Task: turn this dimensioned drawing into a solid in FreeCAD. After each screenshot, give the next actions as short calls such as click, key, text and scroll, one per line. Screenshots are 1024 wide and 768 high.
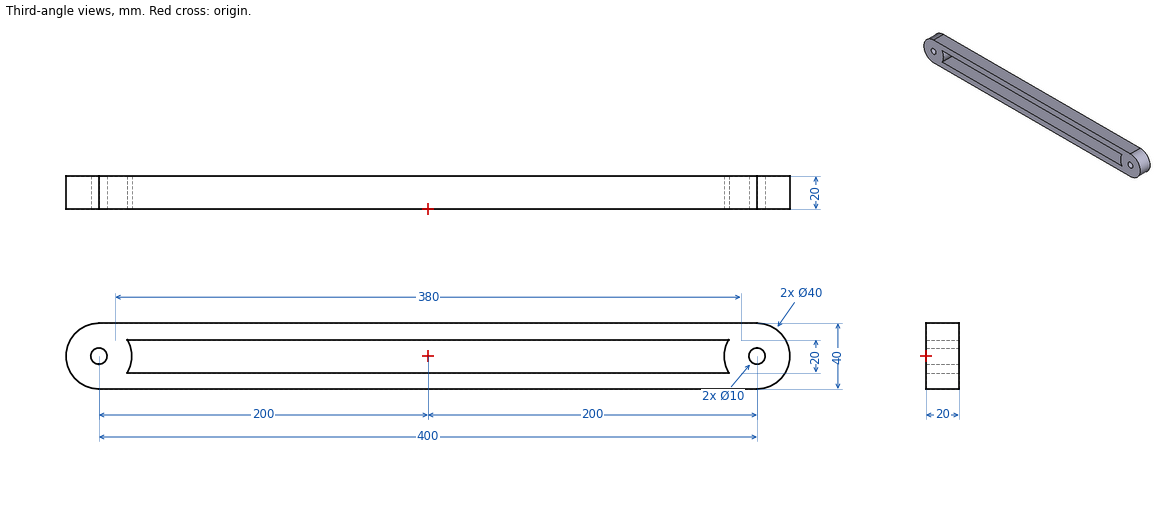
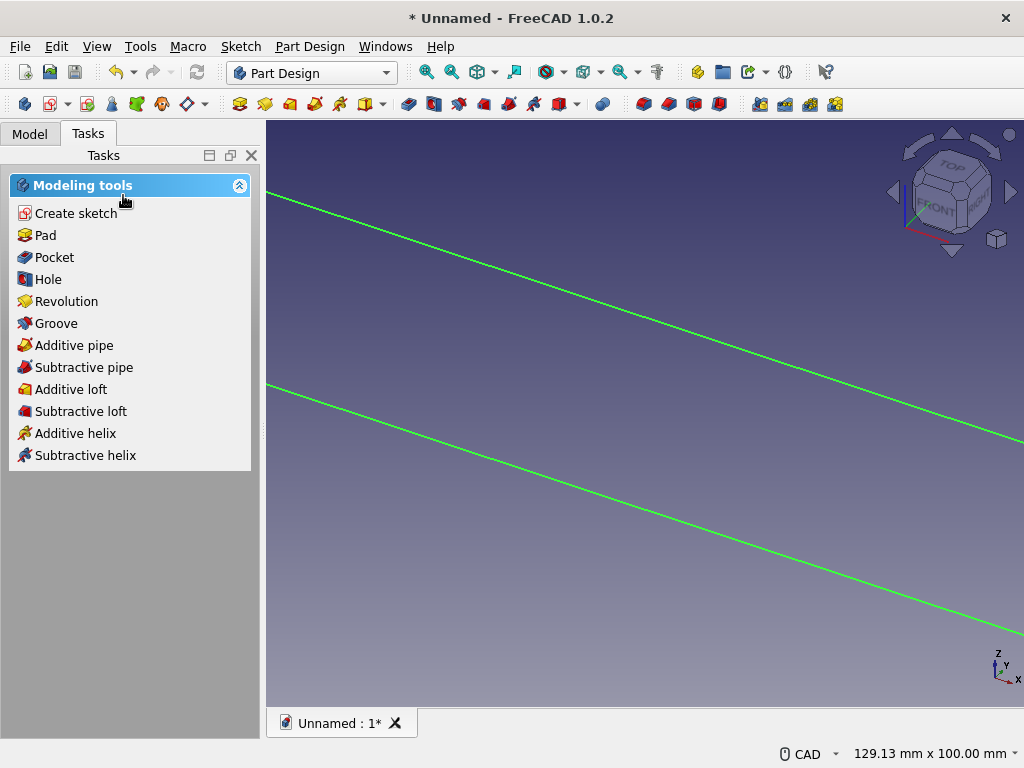
click(240, 104)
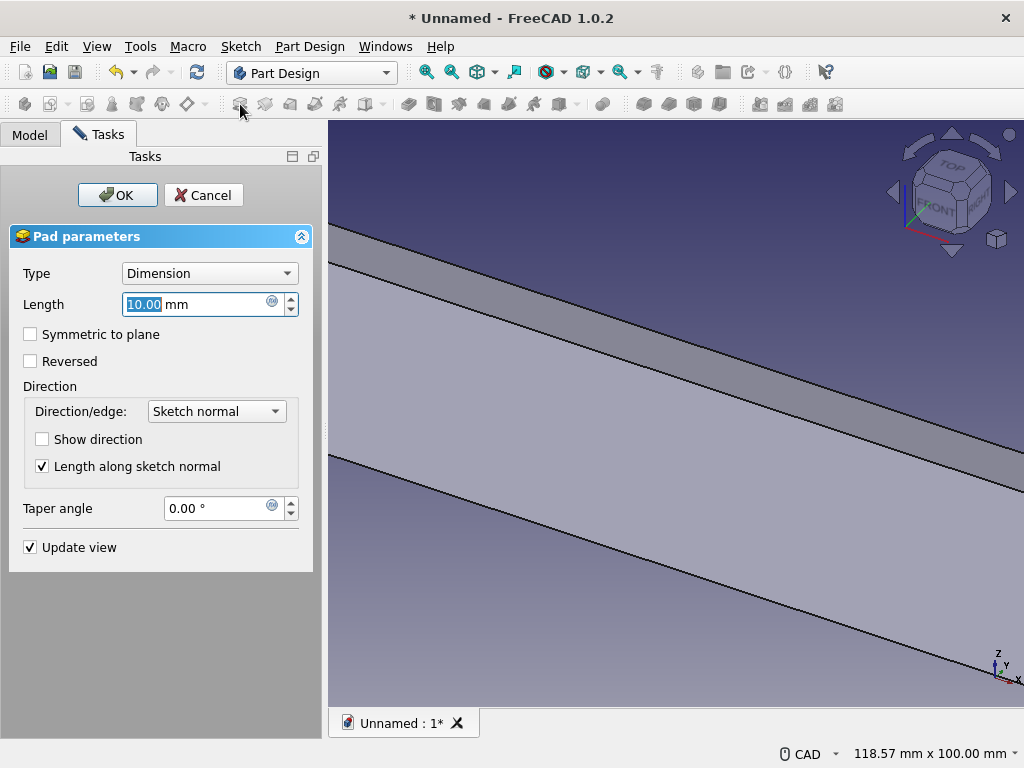
text(20)
key(Tab)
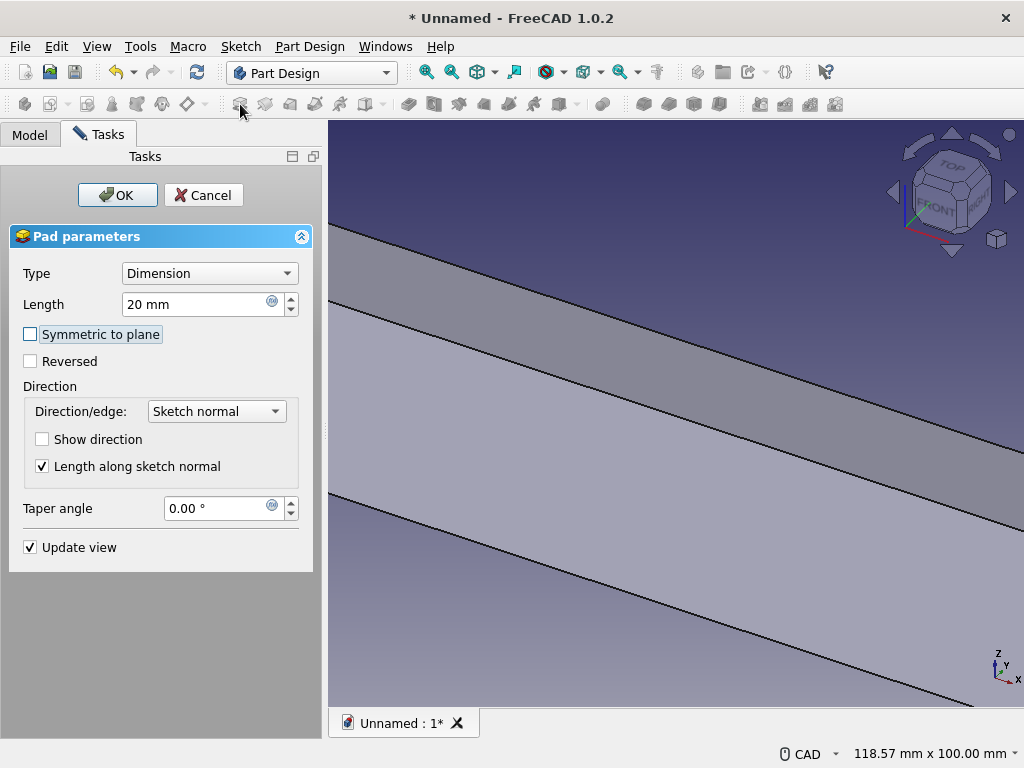
click(31, 361)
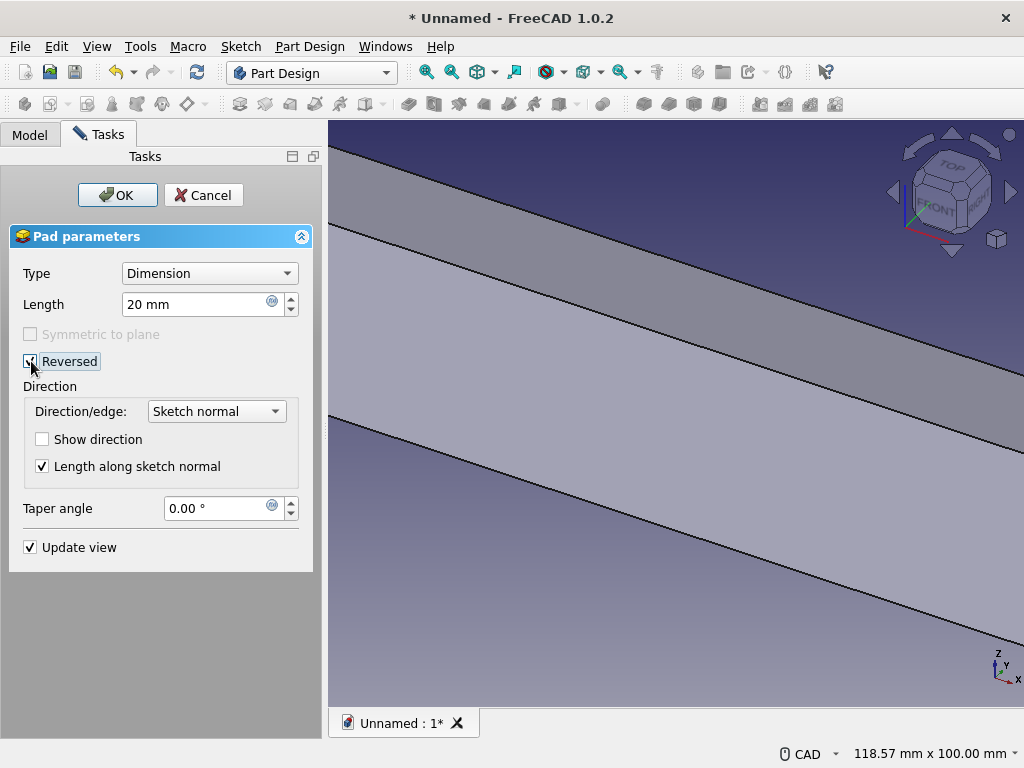
click(118, 195)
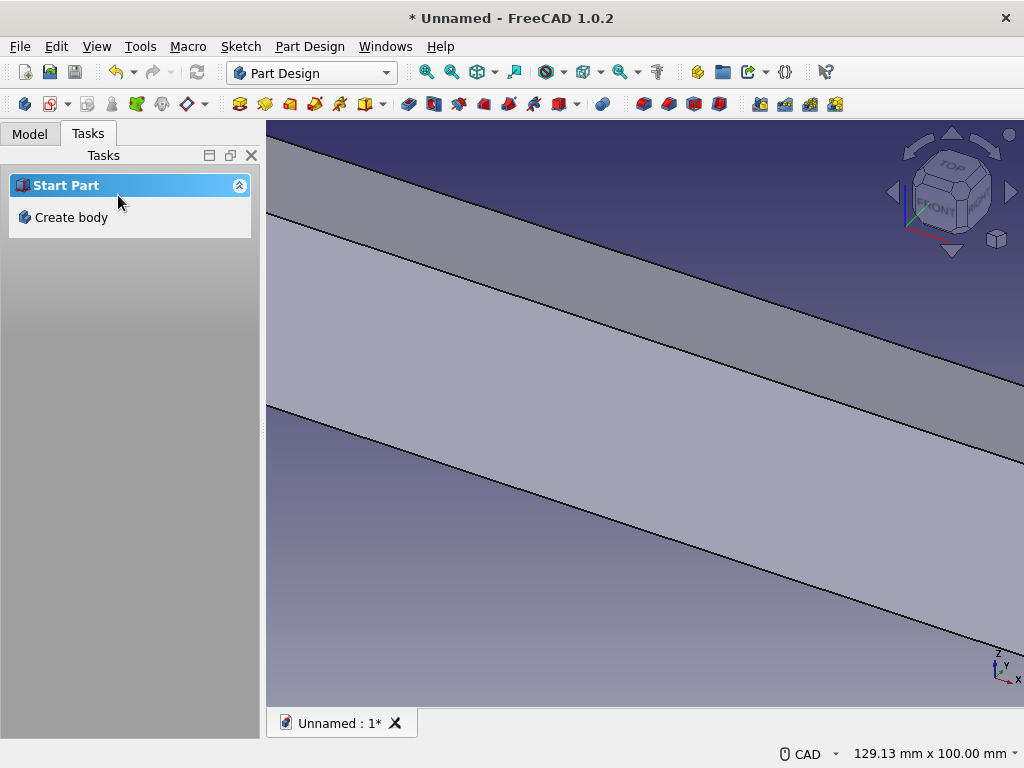
click(427, 72)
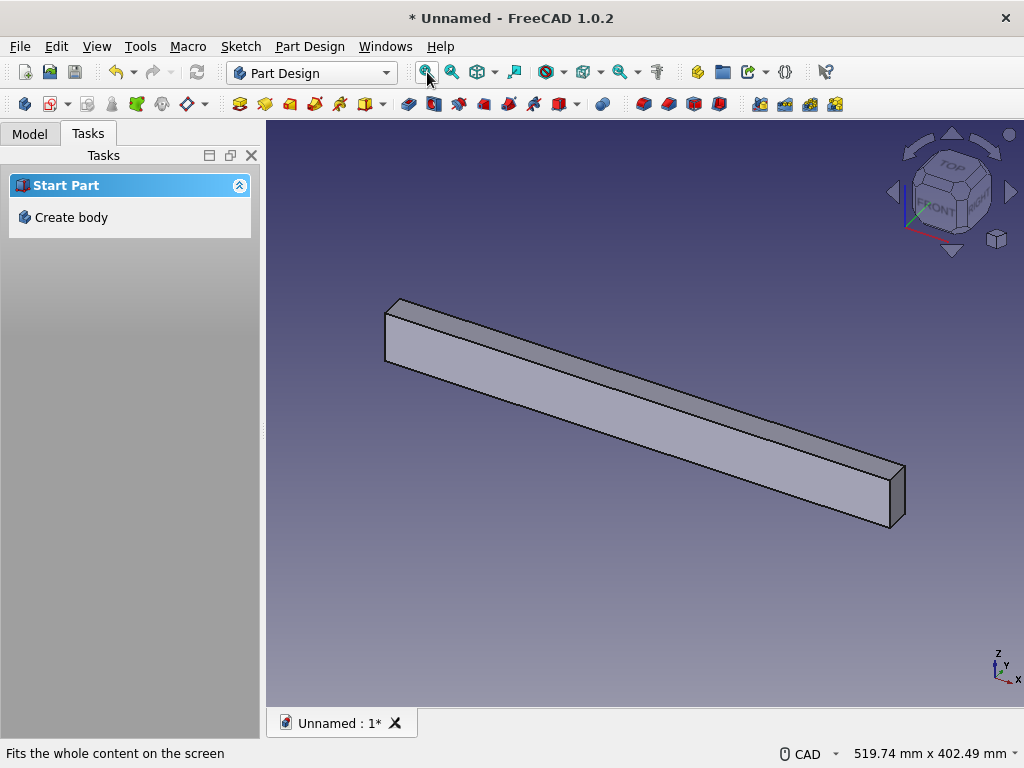
key(4)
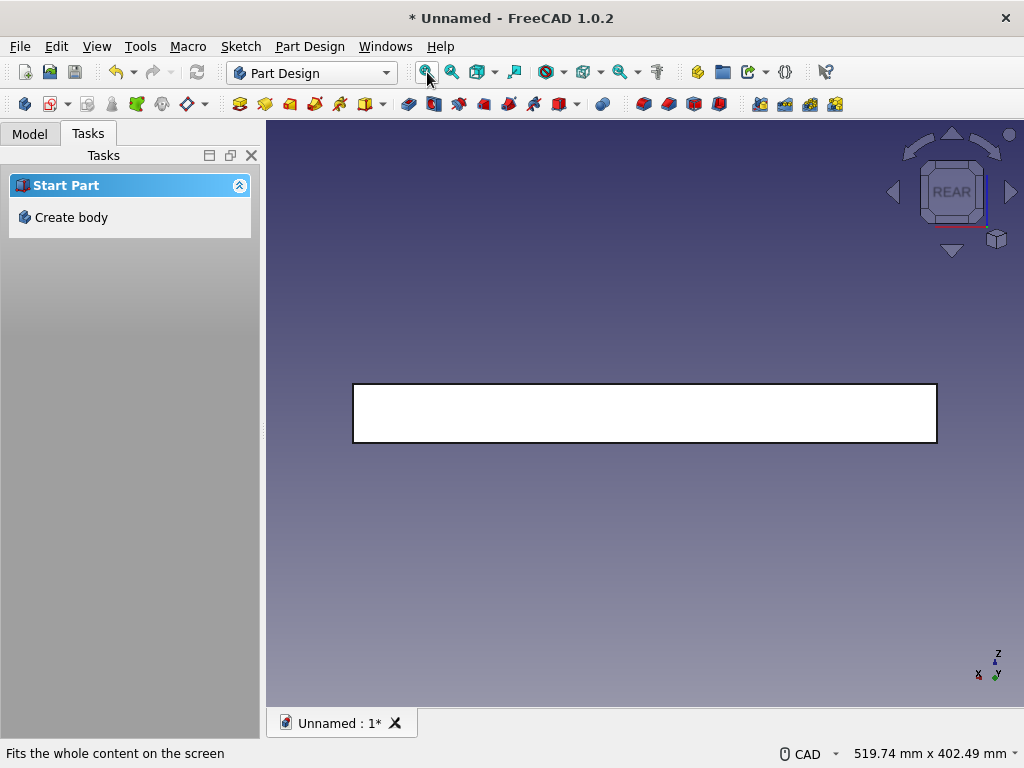
click(395, 413)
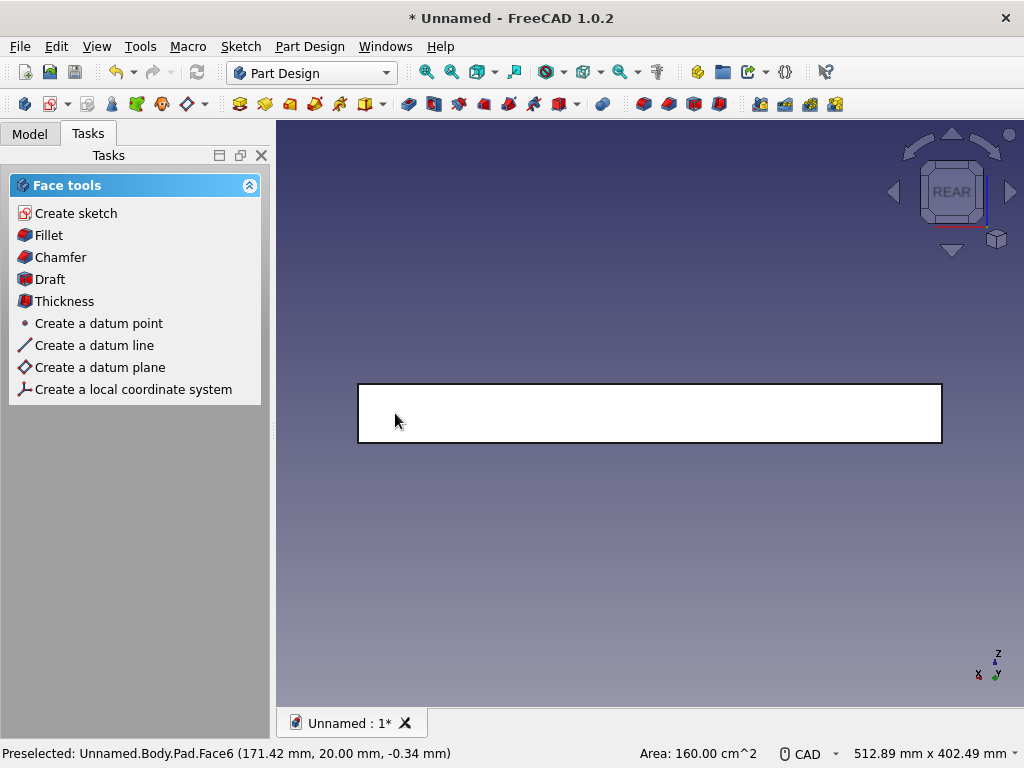
click(50, 104)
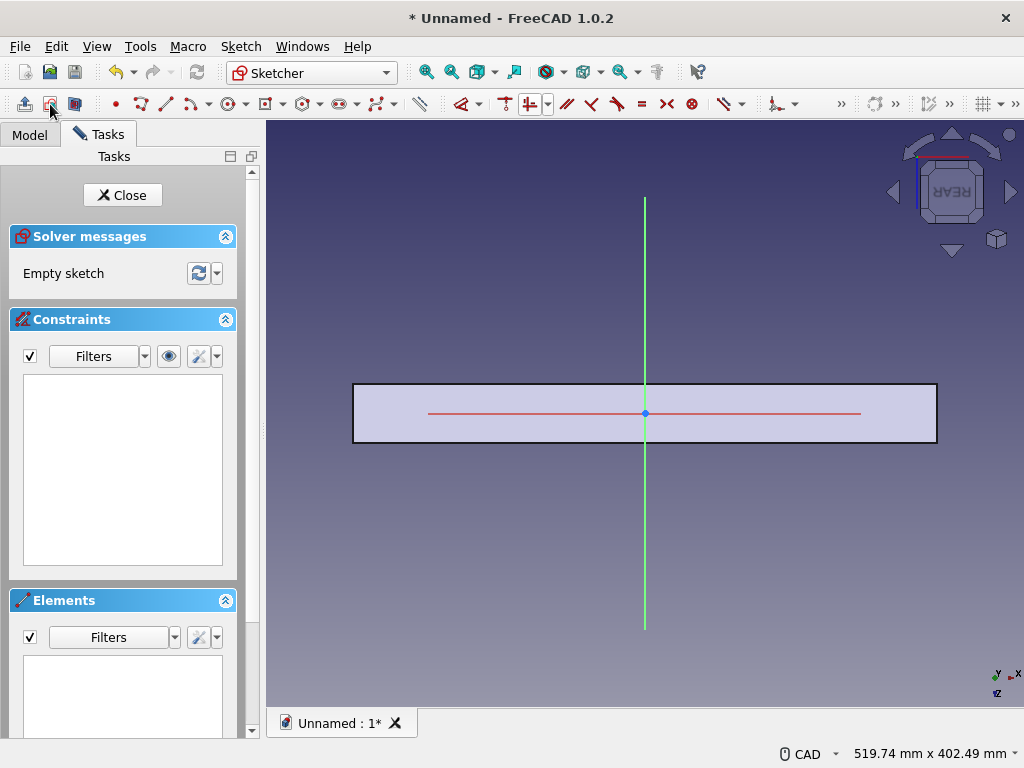
scroll(437, 414, down, 2)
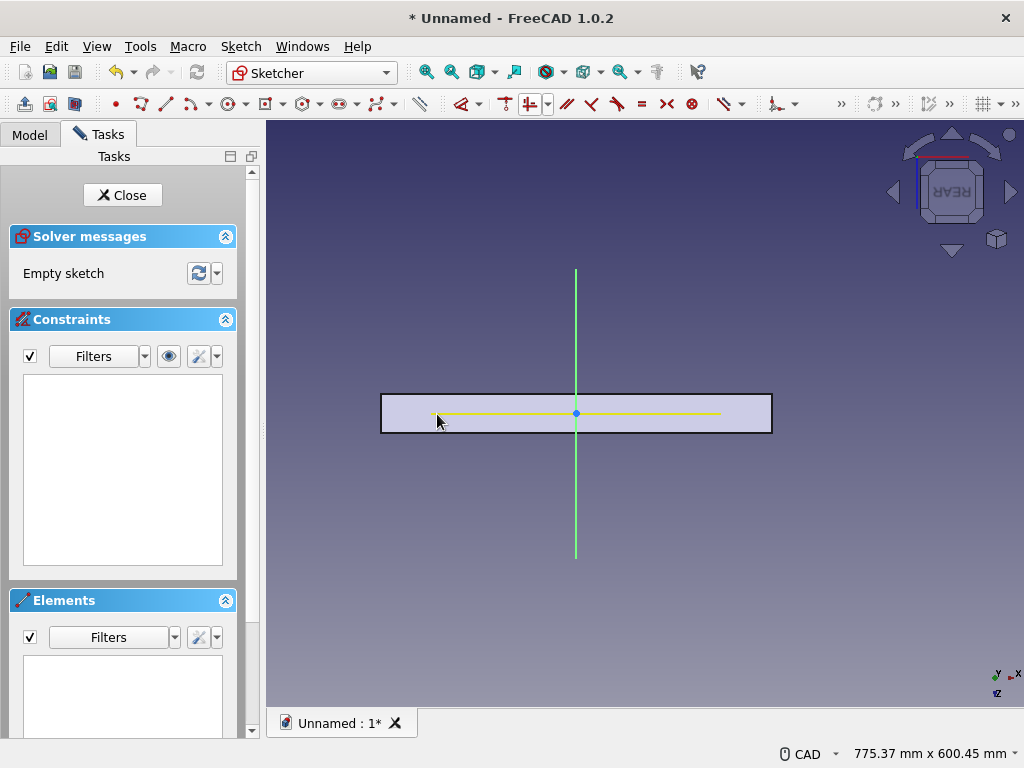
click(264, 104)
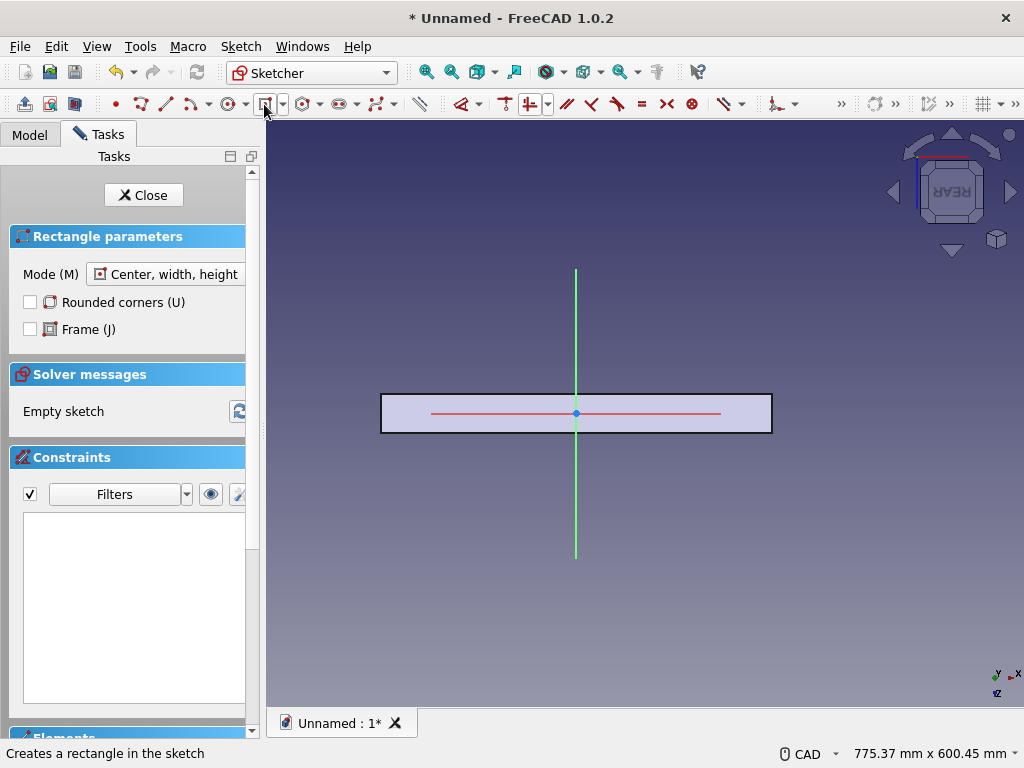
scroll(577, 414, up, 3)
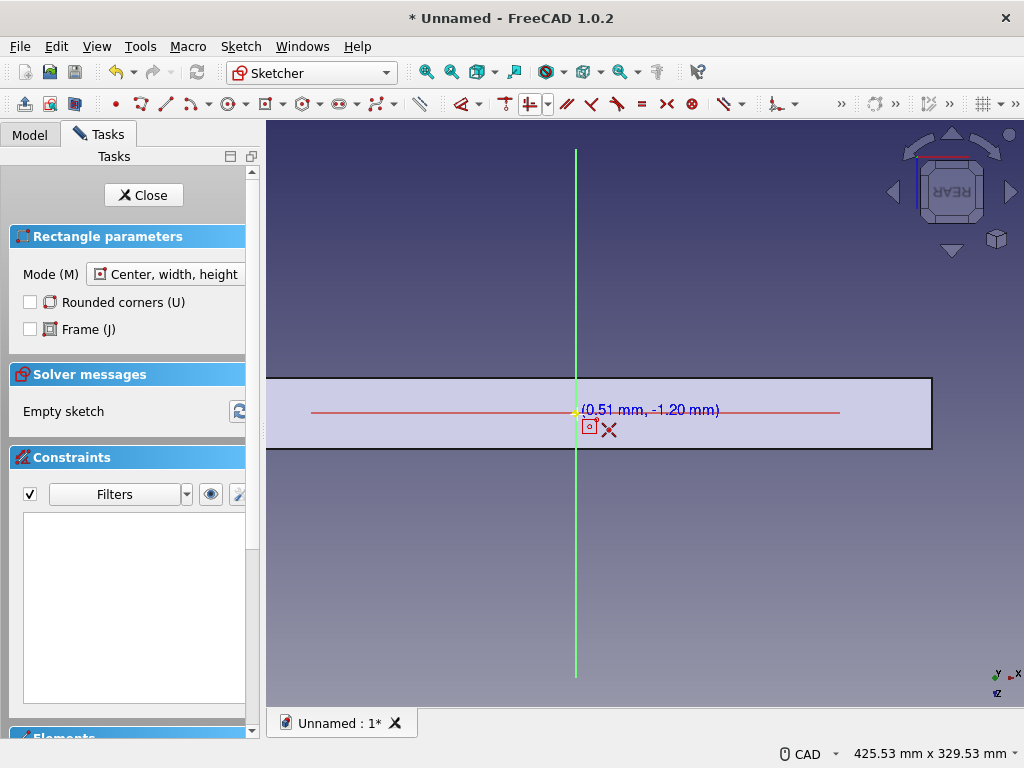
click(576, 413)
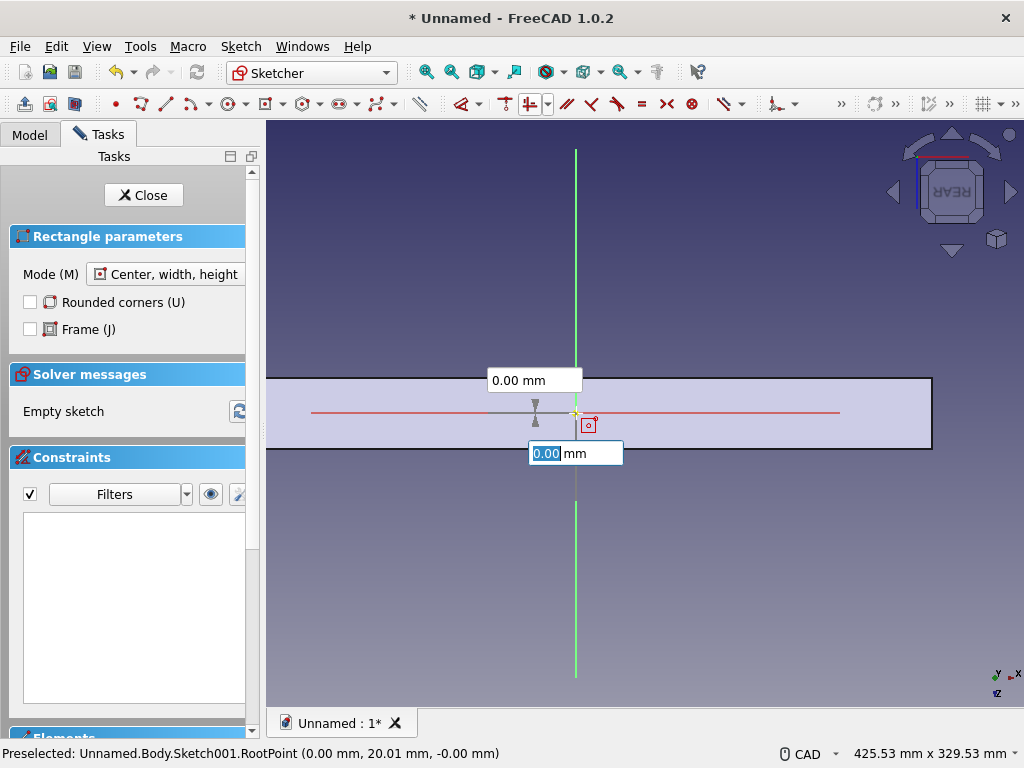
scroll(577, 414, down, 3)